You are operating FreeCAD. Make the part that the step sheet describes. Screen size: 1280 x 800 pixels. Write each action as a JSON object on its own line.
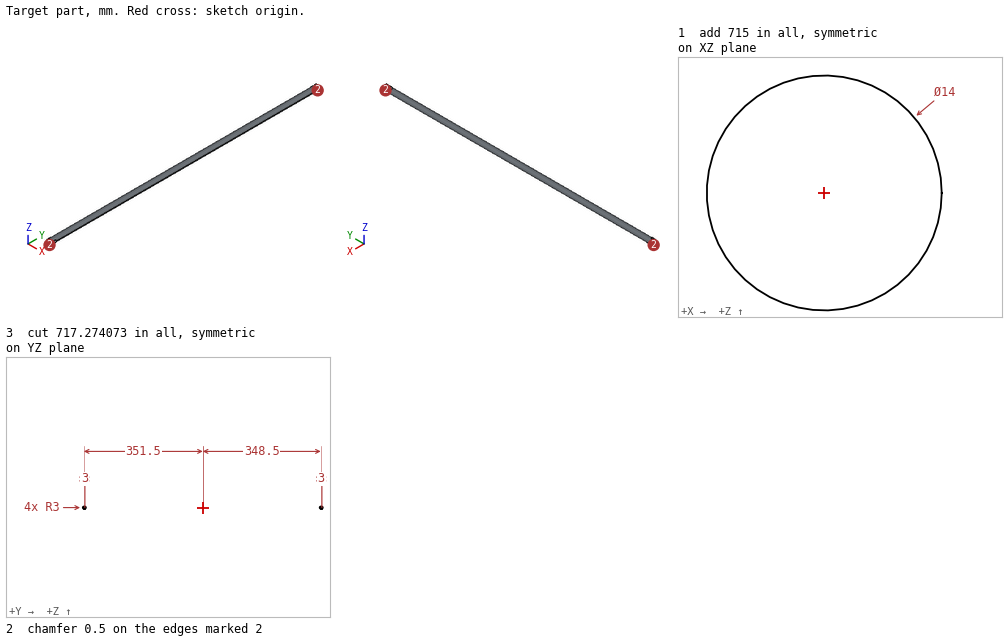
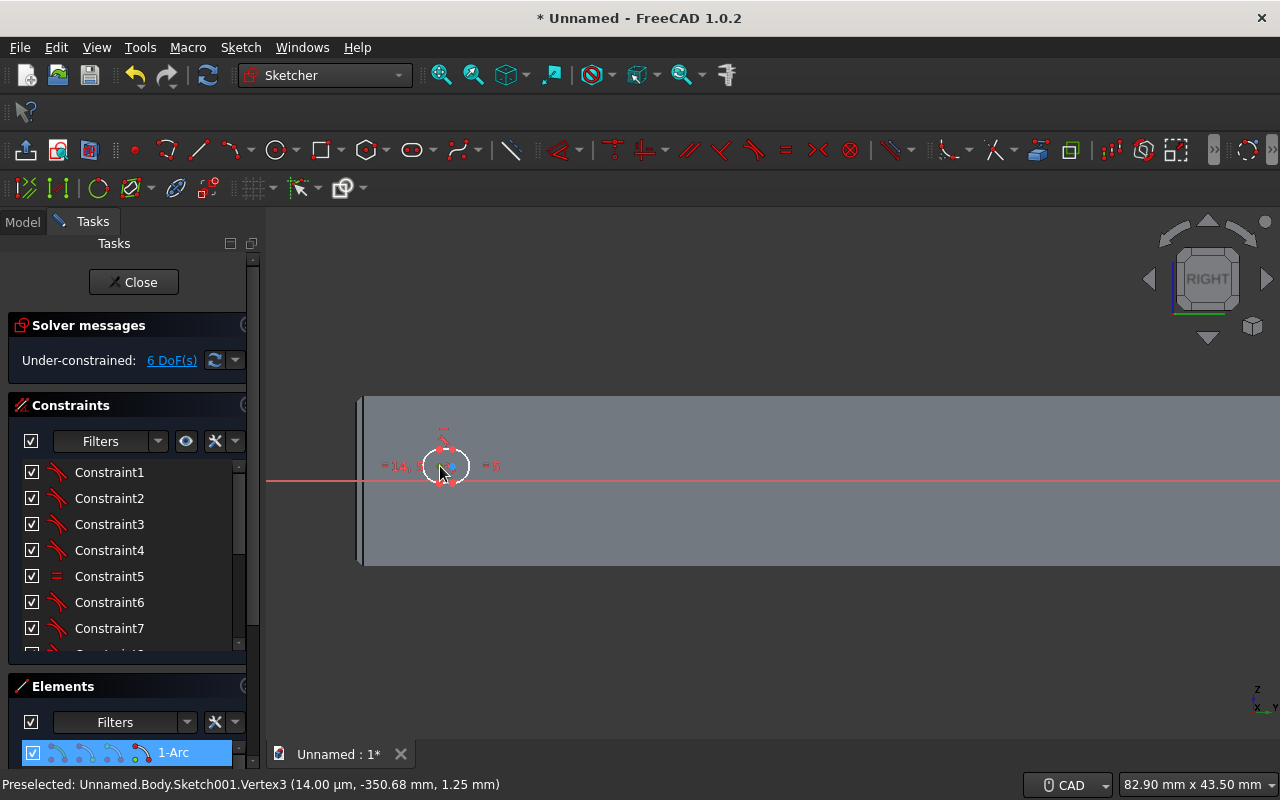
{"action": "left_click", "coordinate": [353, 481]}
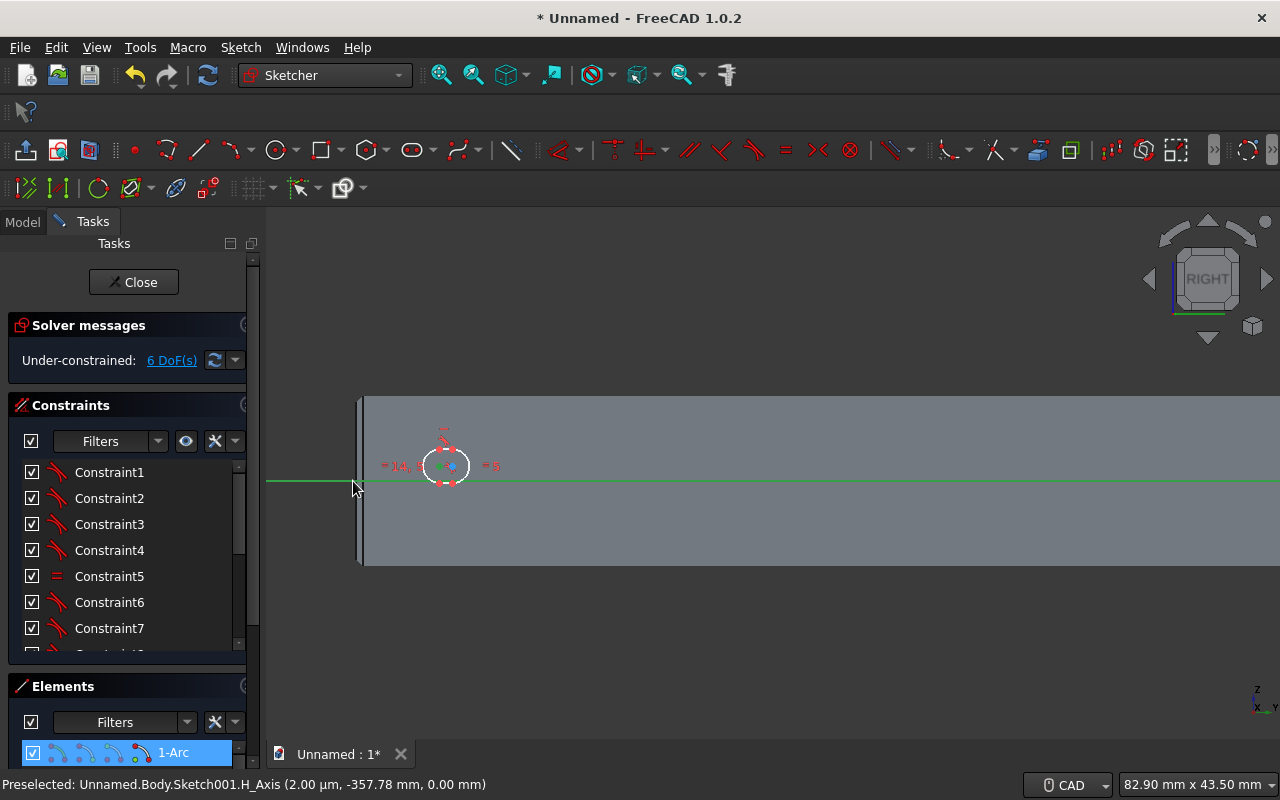
{"action": "left_click", "coordinate": [614, 150]}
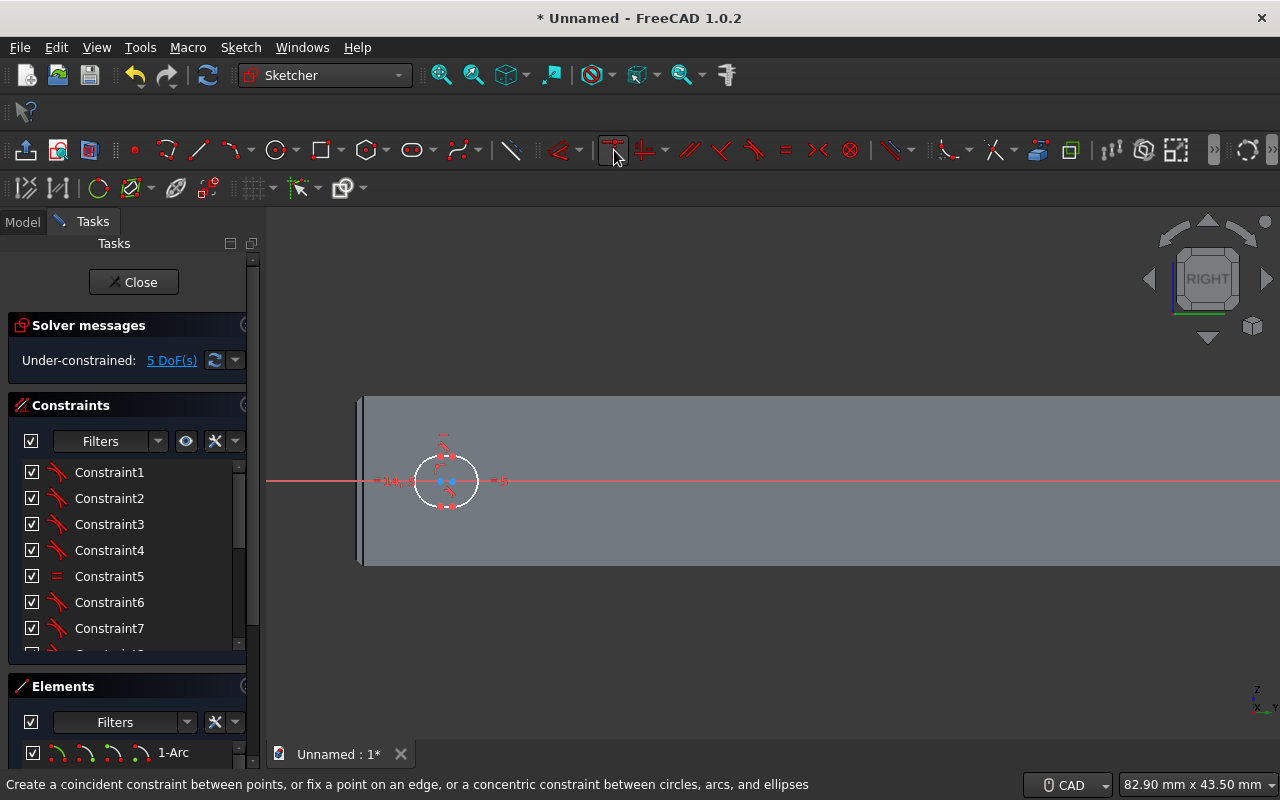
{"action": "left_click", "coordinate": [420, 467]}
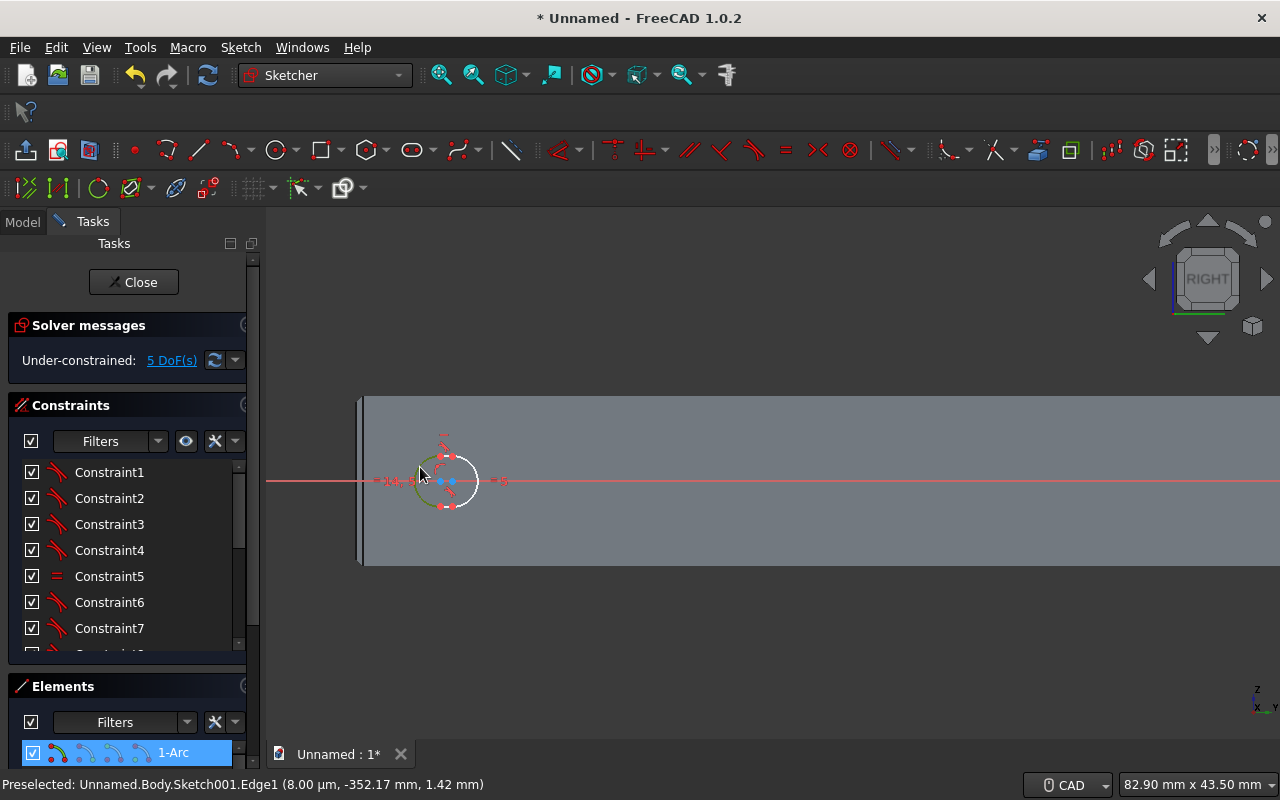
{"action": "left_click", "coordinate": [582, 150]}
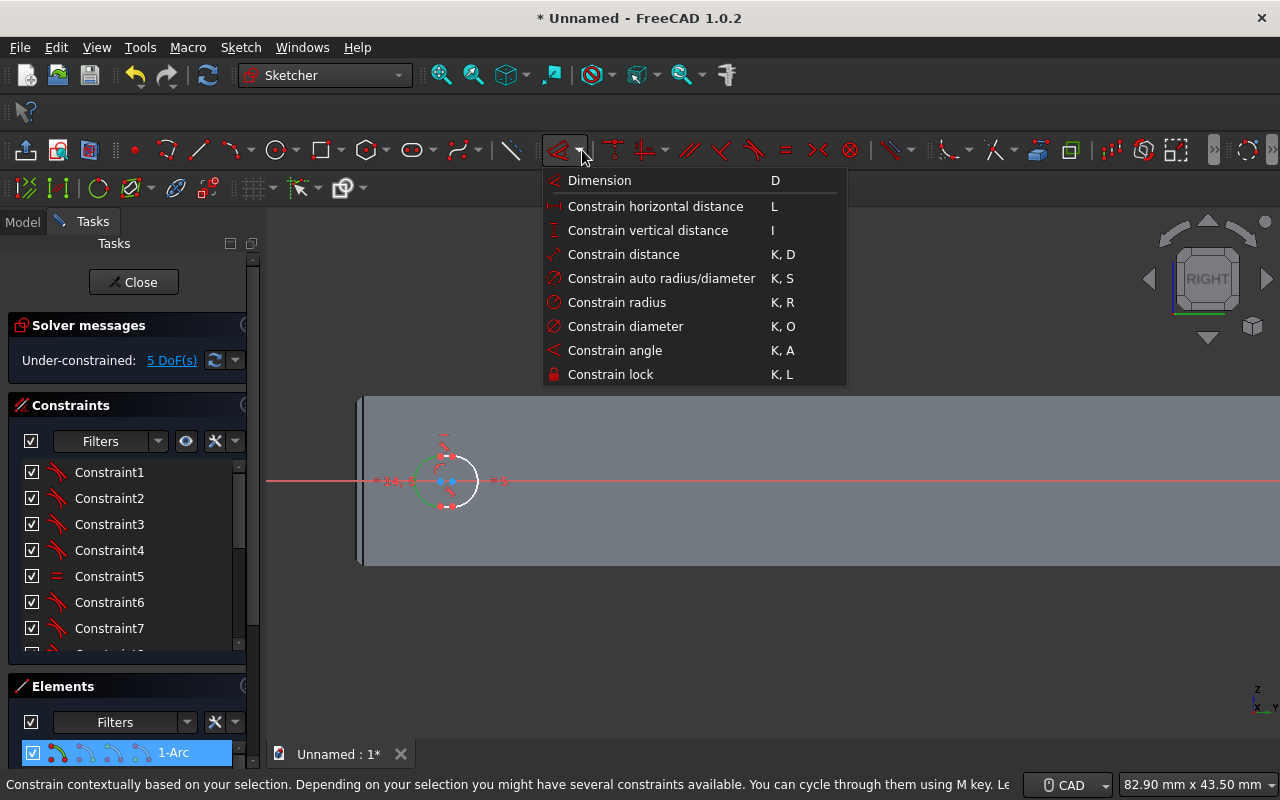
{"action": "left_click", "coordinate": [695, 302]}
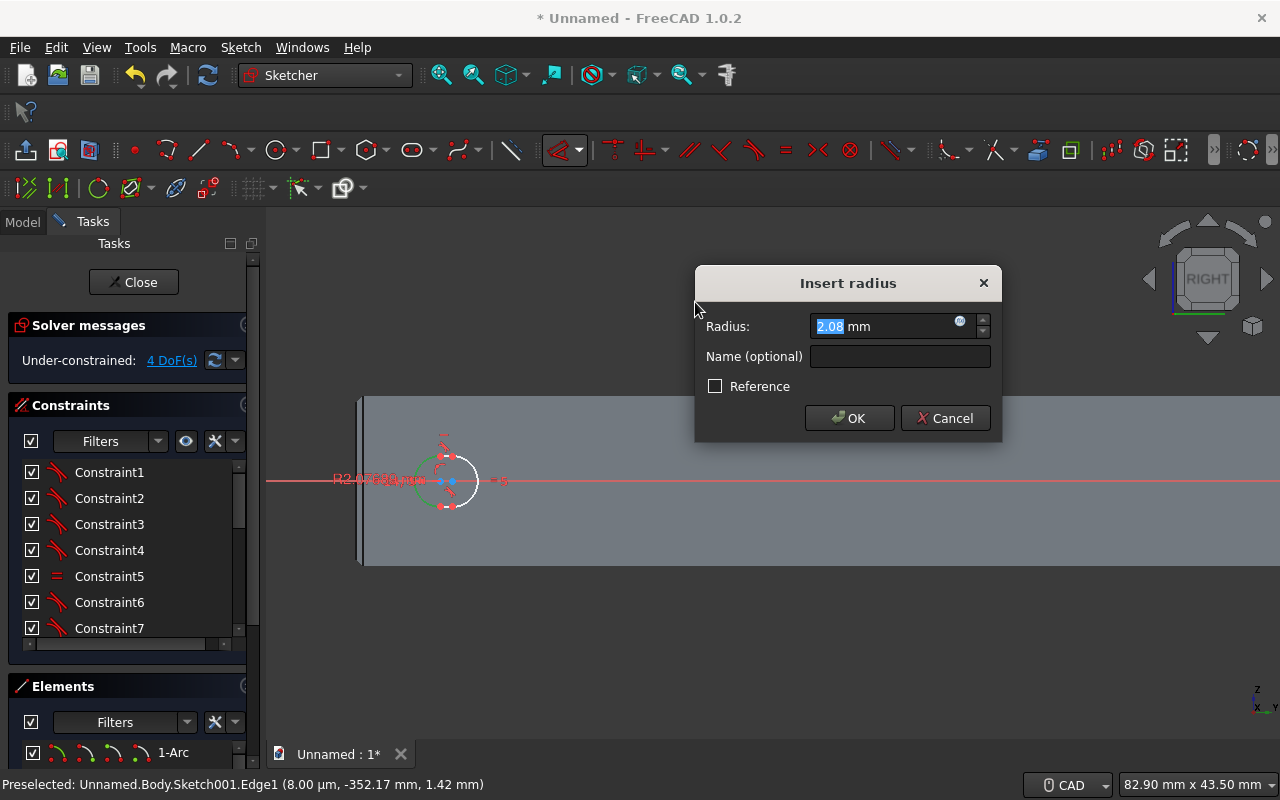
{"action": "type", "text": "3"}
{"action": "key", "text": "Return"}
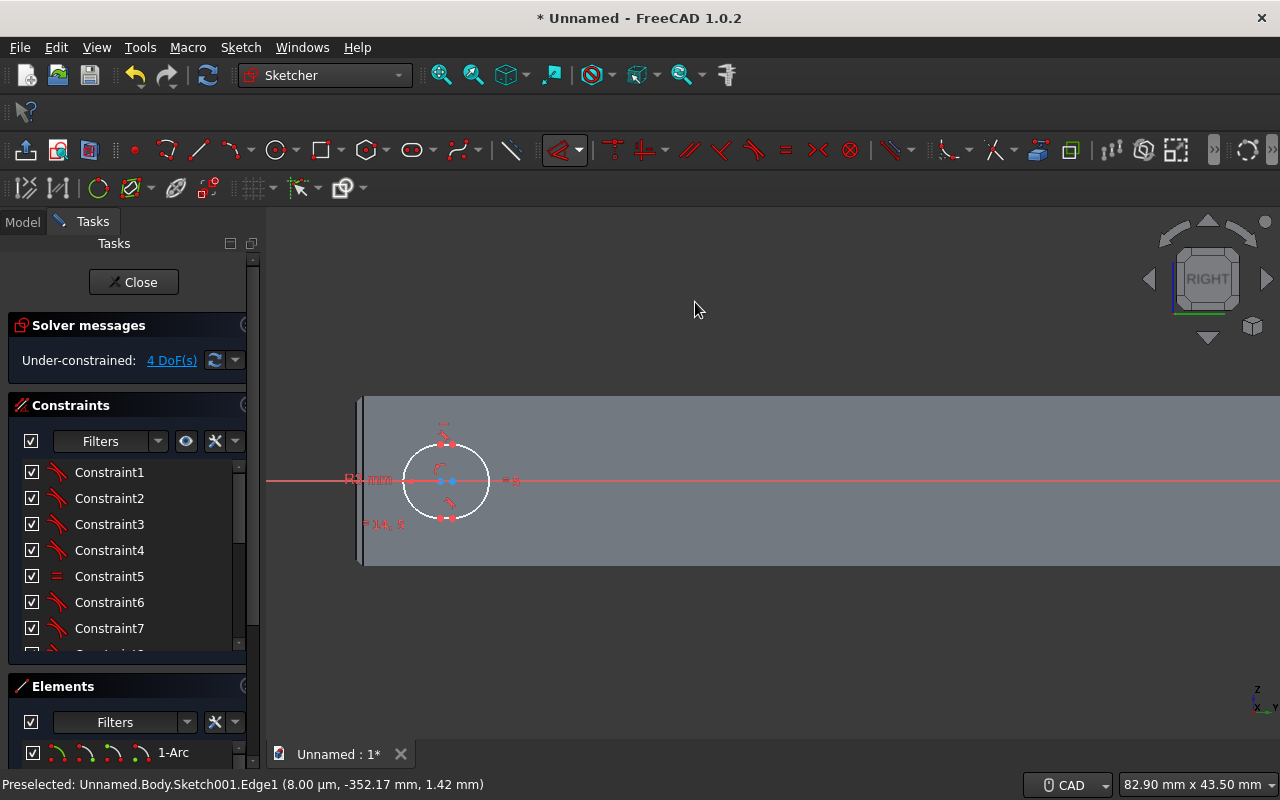
{"action": "left_click", "coordinate": [446, 445]}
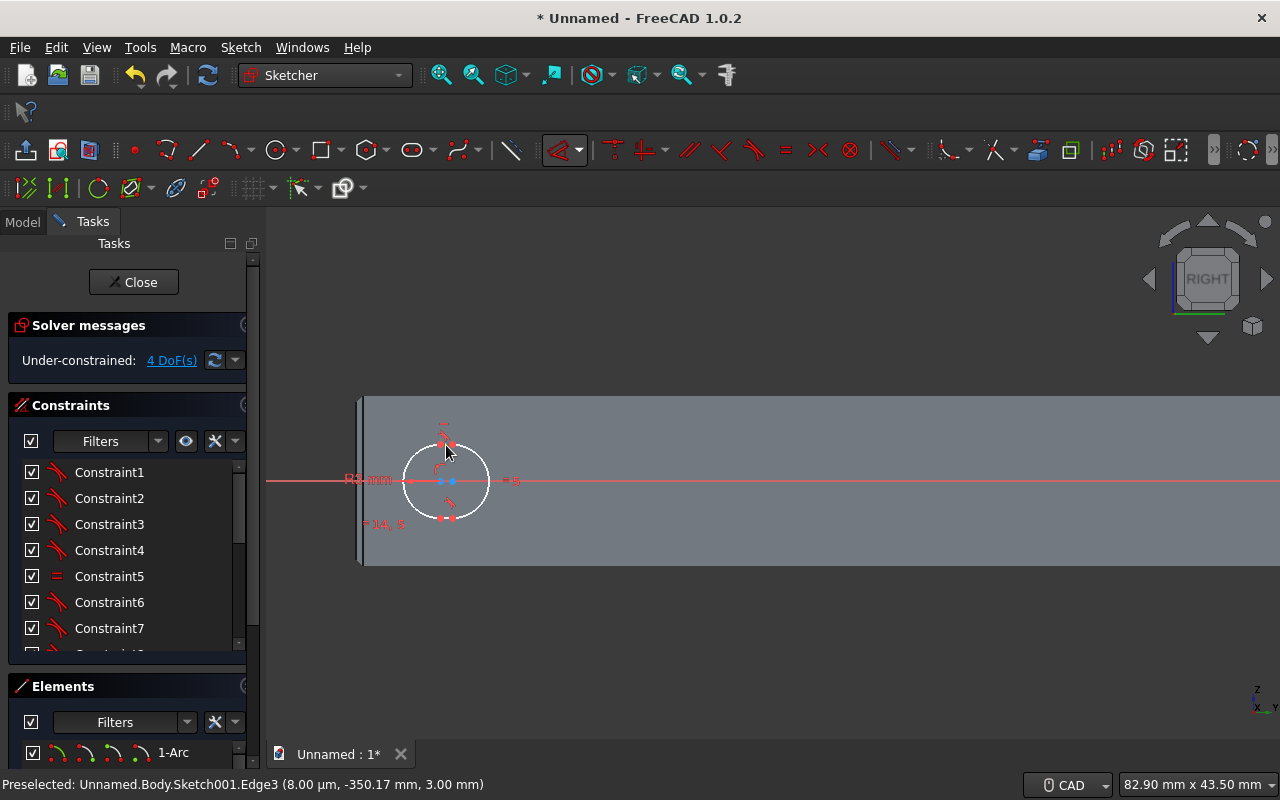
{"action": "left_click", "coordinate": [582, 150]}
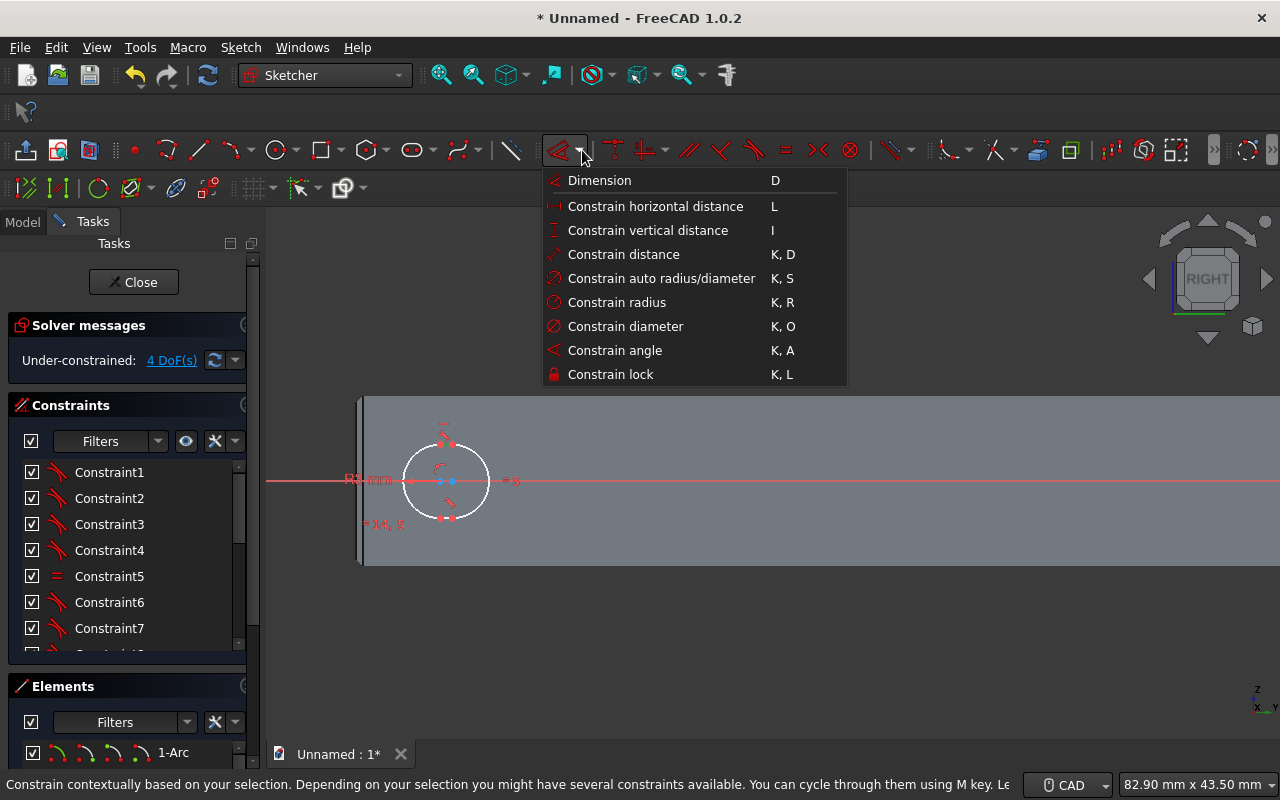
{"action": "left_click", "coordinate": [695, 206]}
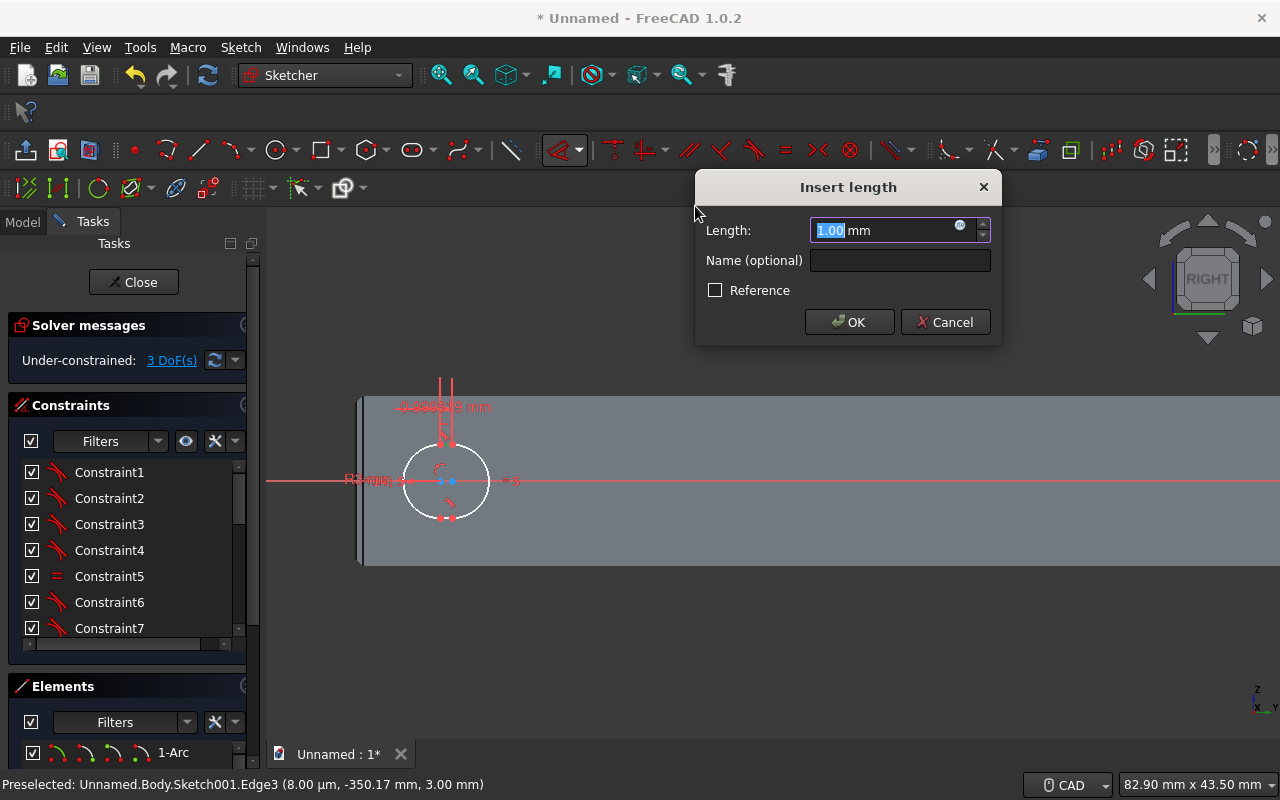
{"action": "type", "text": "3"}
{"action": "key", "text": "Return"}